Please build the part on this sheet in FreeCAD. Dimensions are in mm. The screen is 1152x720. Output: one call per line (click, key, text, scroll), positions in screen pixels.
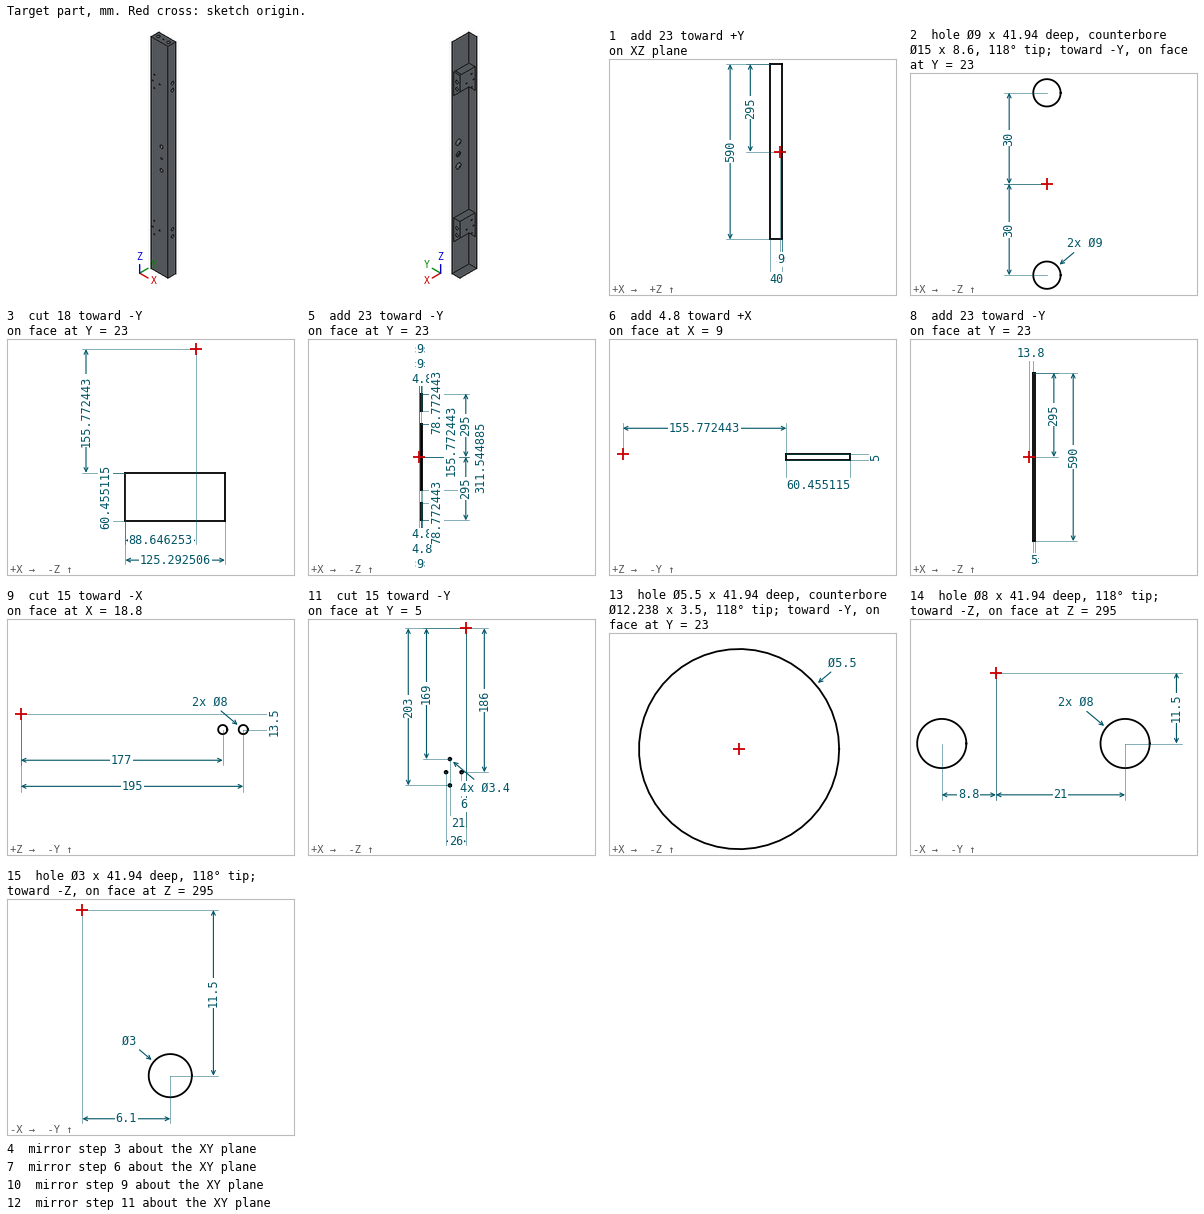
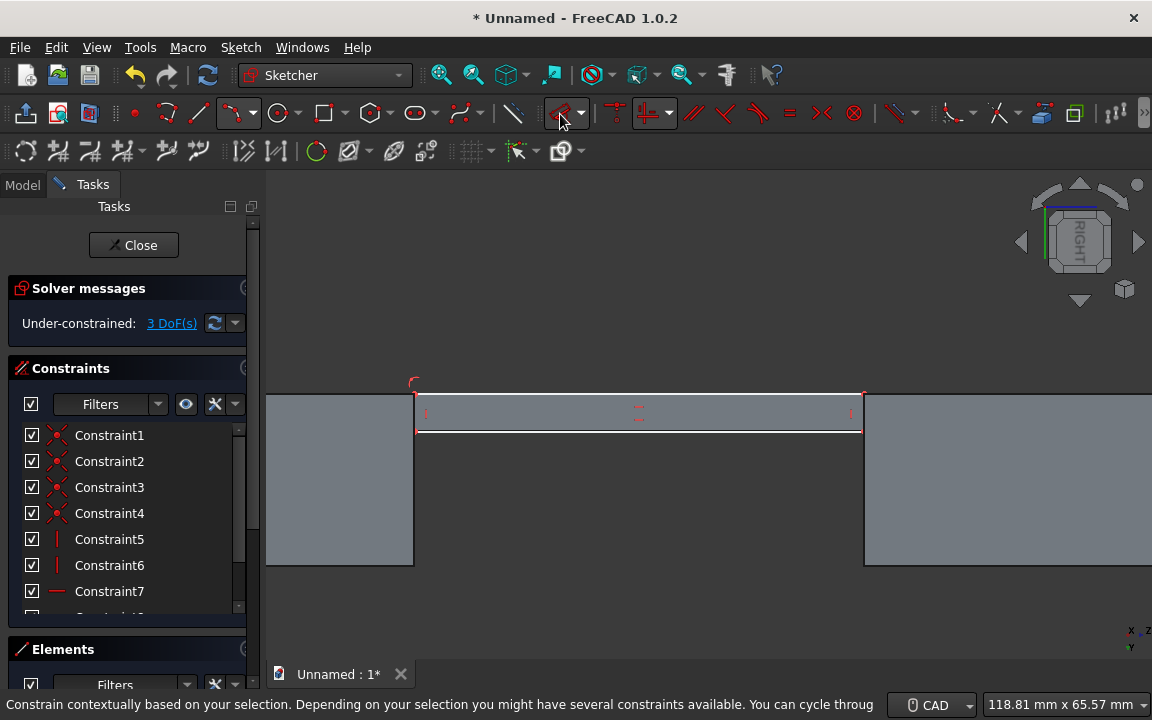
click(414, 405)
click(380, 413)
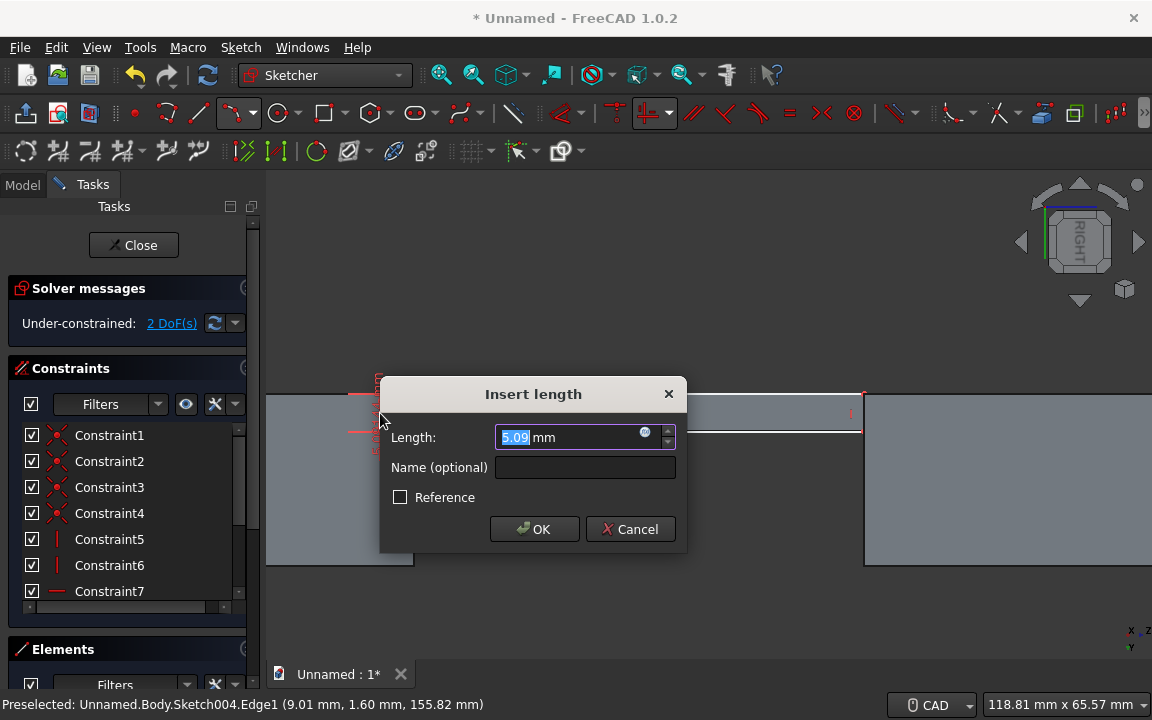
text(5)
key(Return)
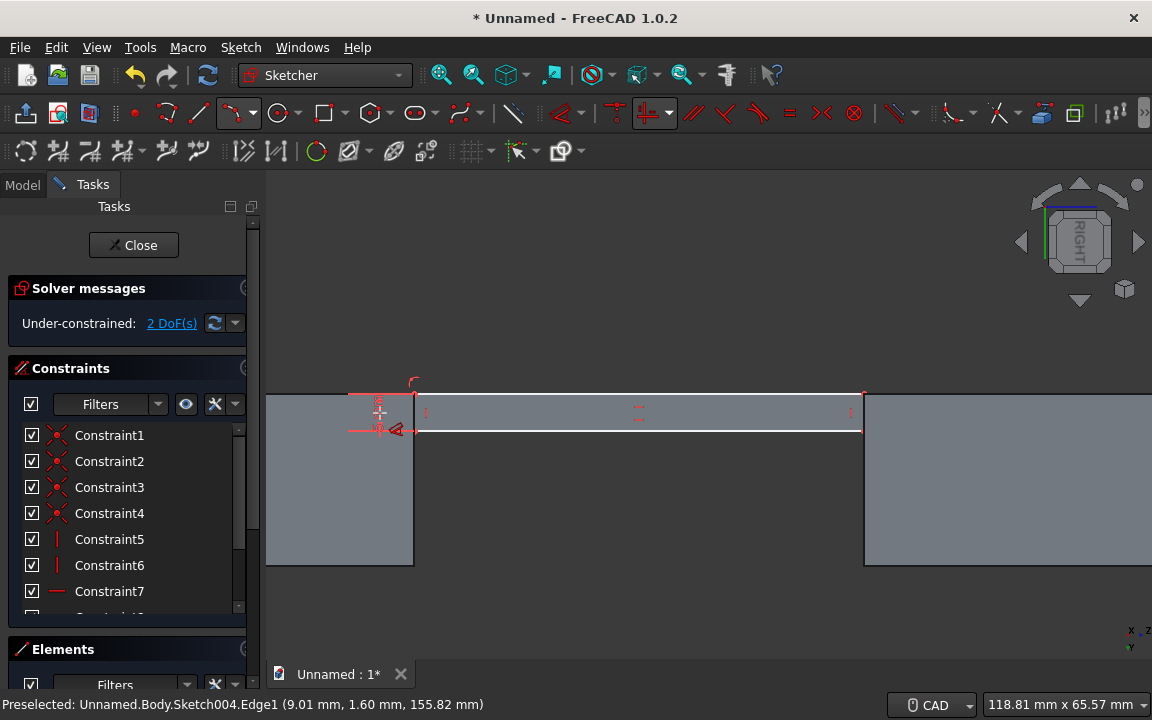
click(549, 431)
click(639, 465)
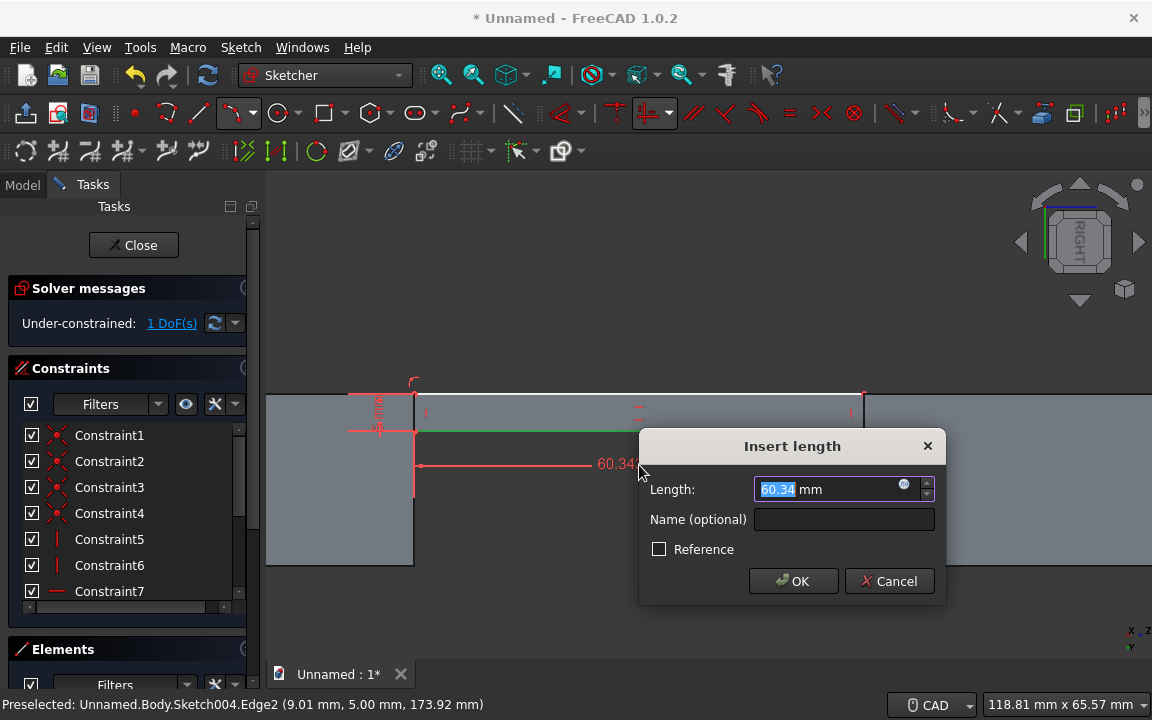
text(60.455115)
key(Return)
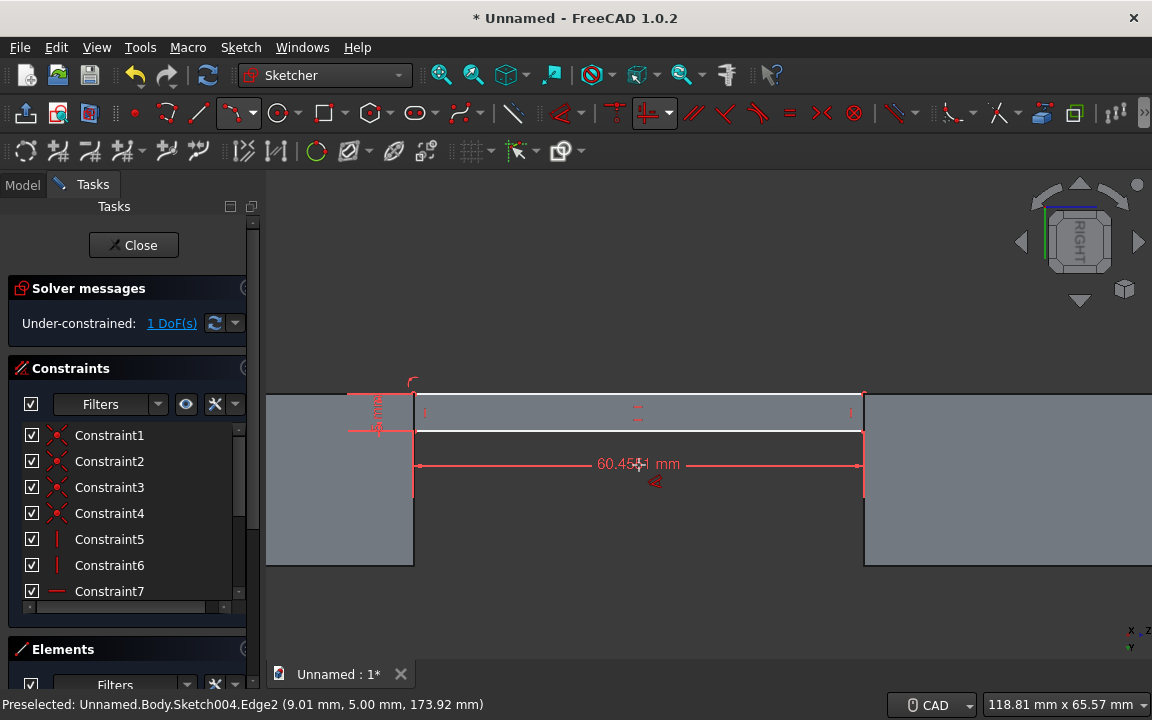
click(413, 394)
click(354, 360)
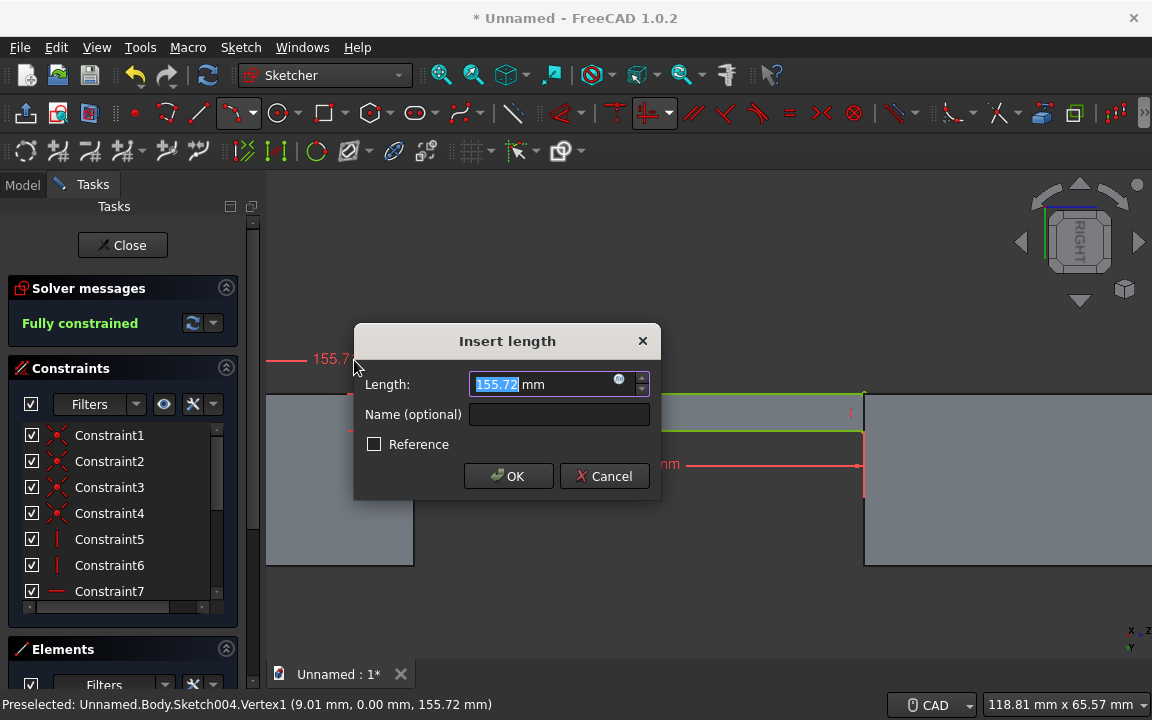
text(155.772443)
key(Return)
key(Escape)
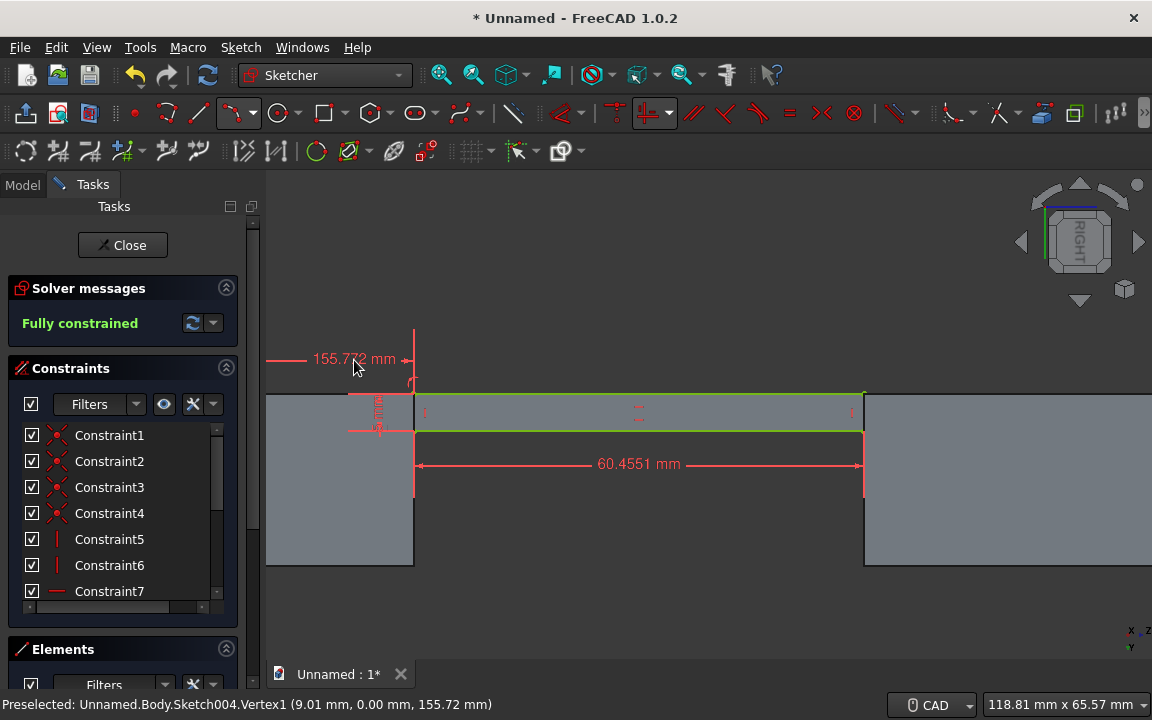
click(123, 245)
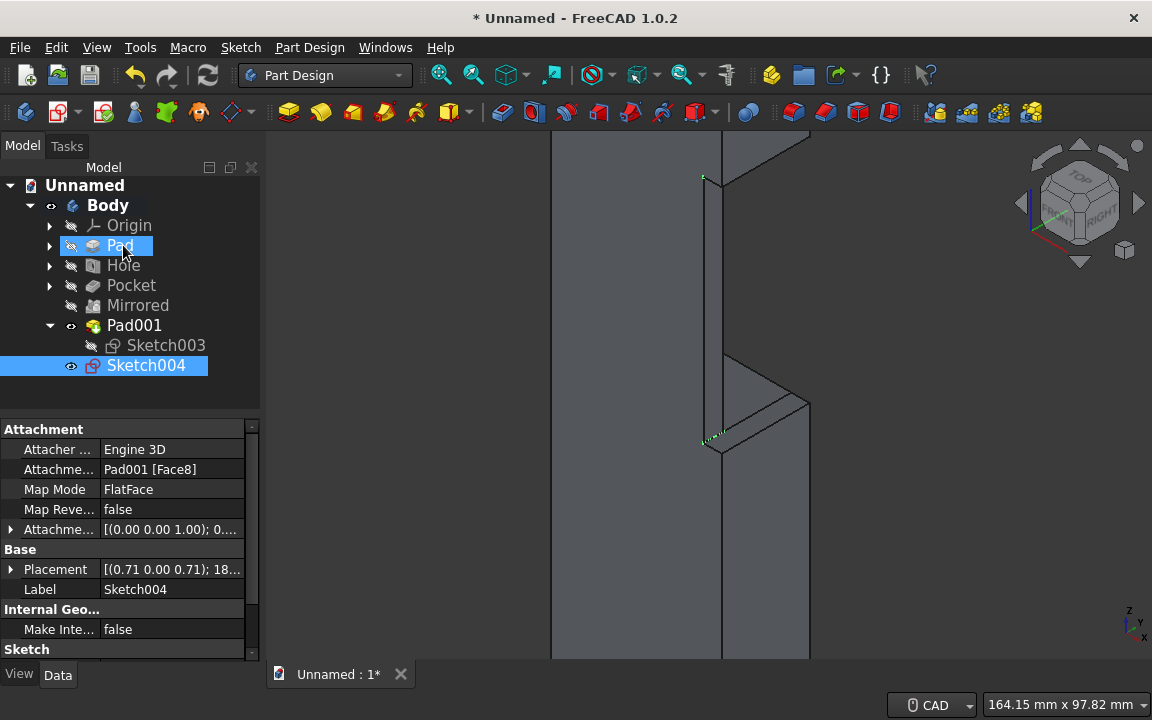
click(290, 112)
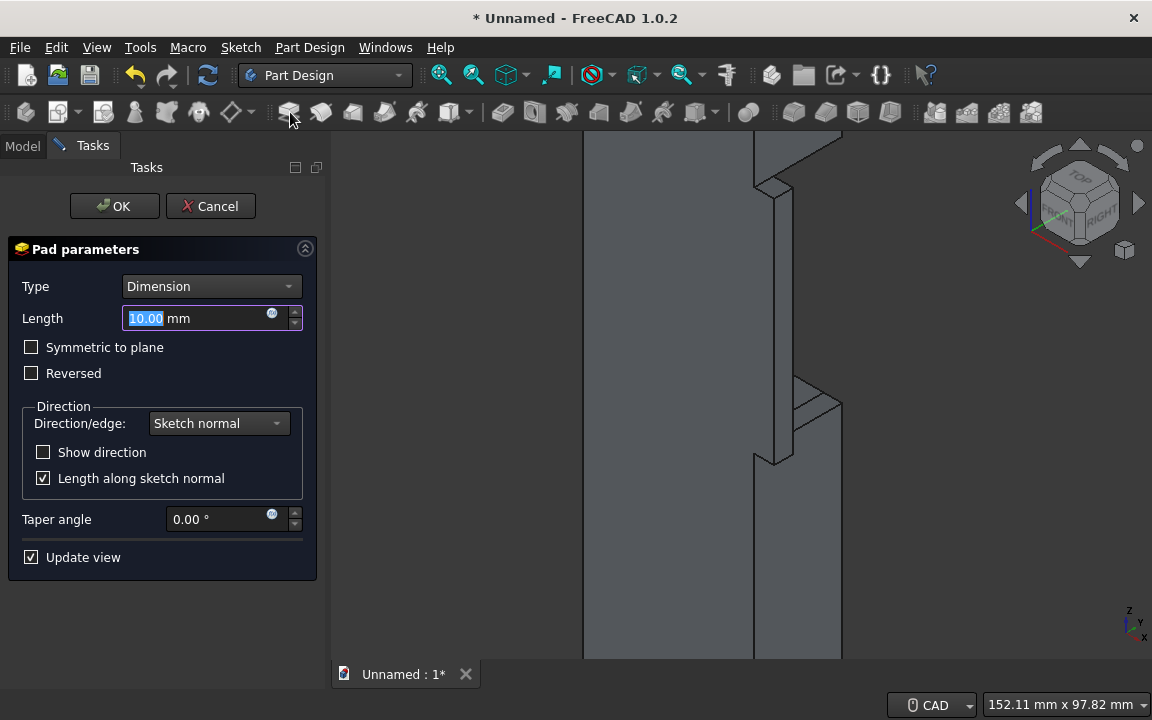
text(4.8)
key(Tab)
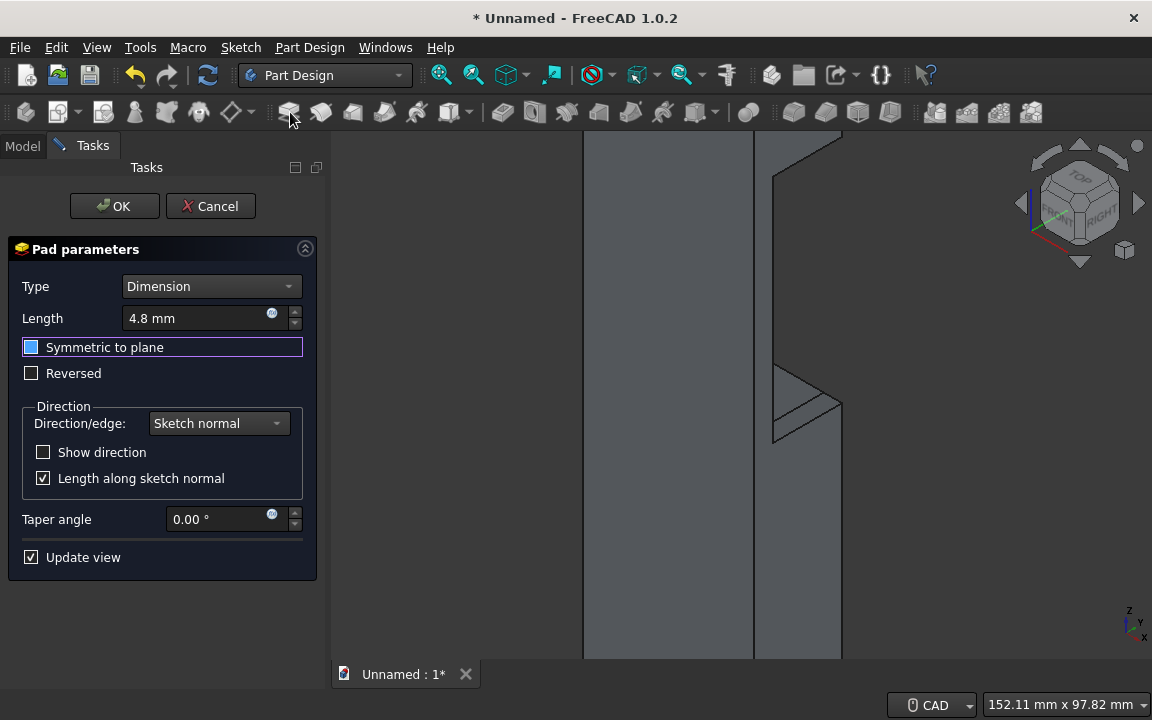
click(115, 206)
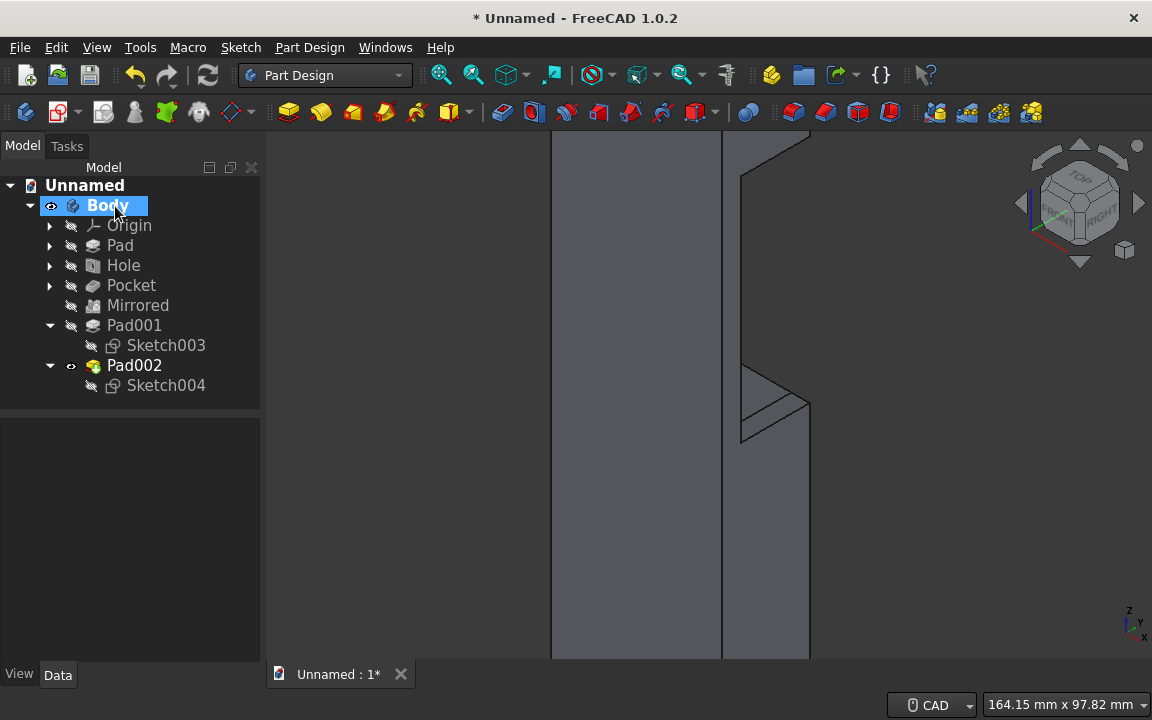
click(442, 76)